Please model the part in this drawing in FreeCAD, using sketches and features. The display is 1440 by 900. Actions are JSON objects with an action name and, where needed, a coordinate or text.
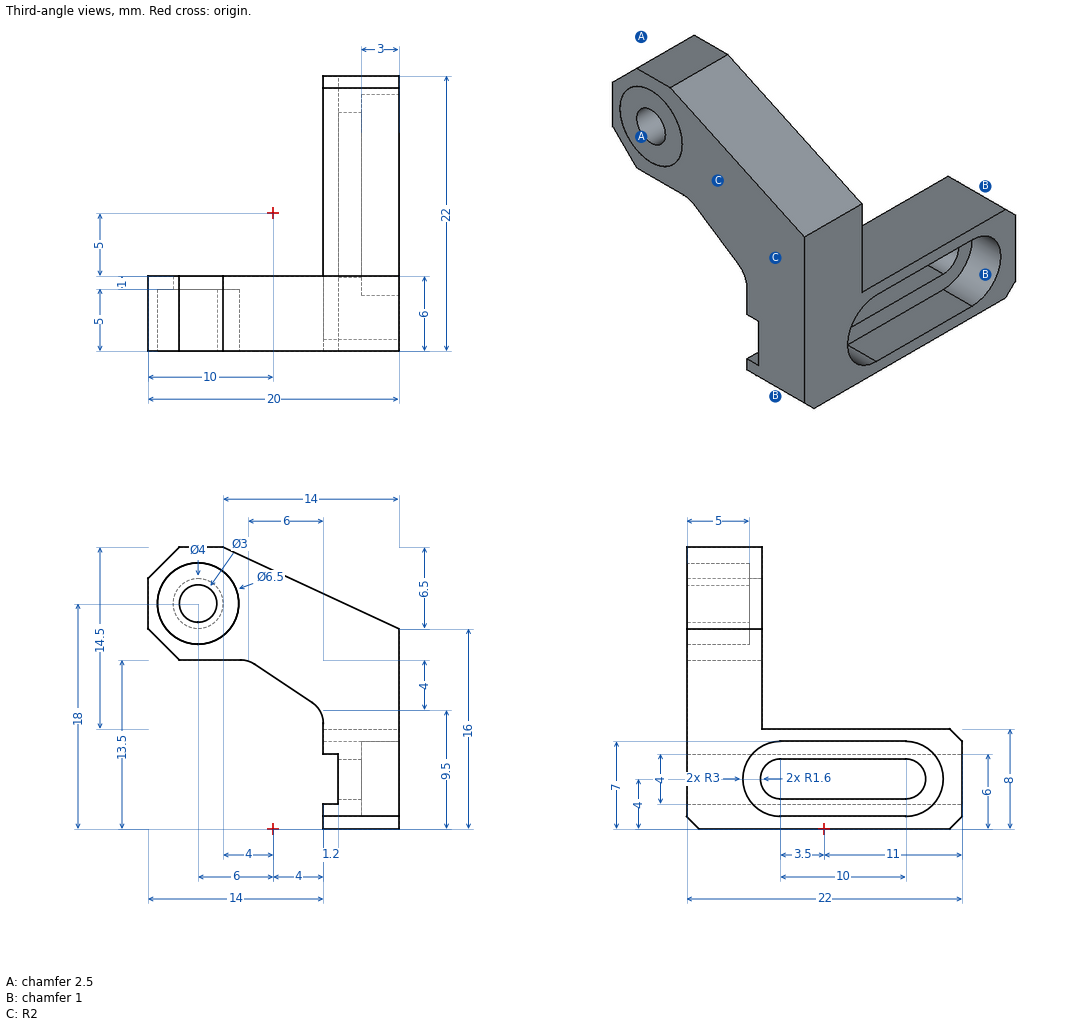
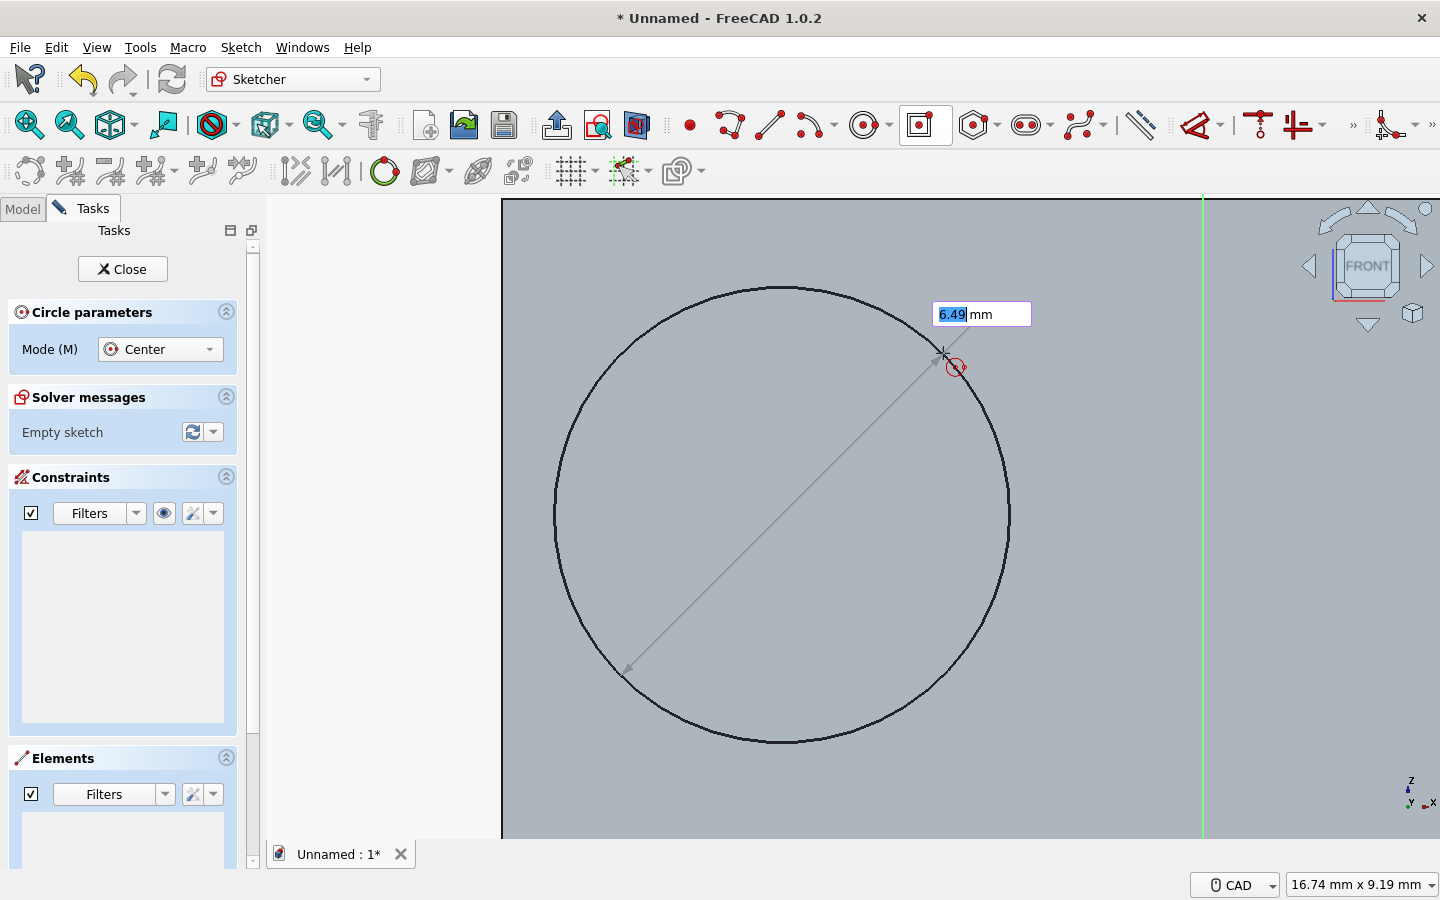
{"action": "type", "text": "6.5"}
{"action": "key", "text": "Return"}
{"action": "key", "text": "Escape"}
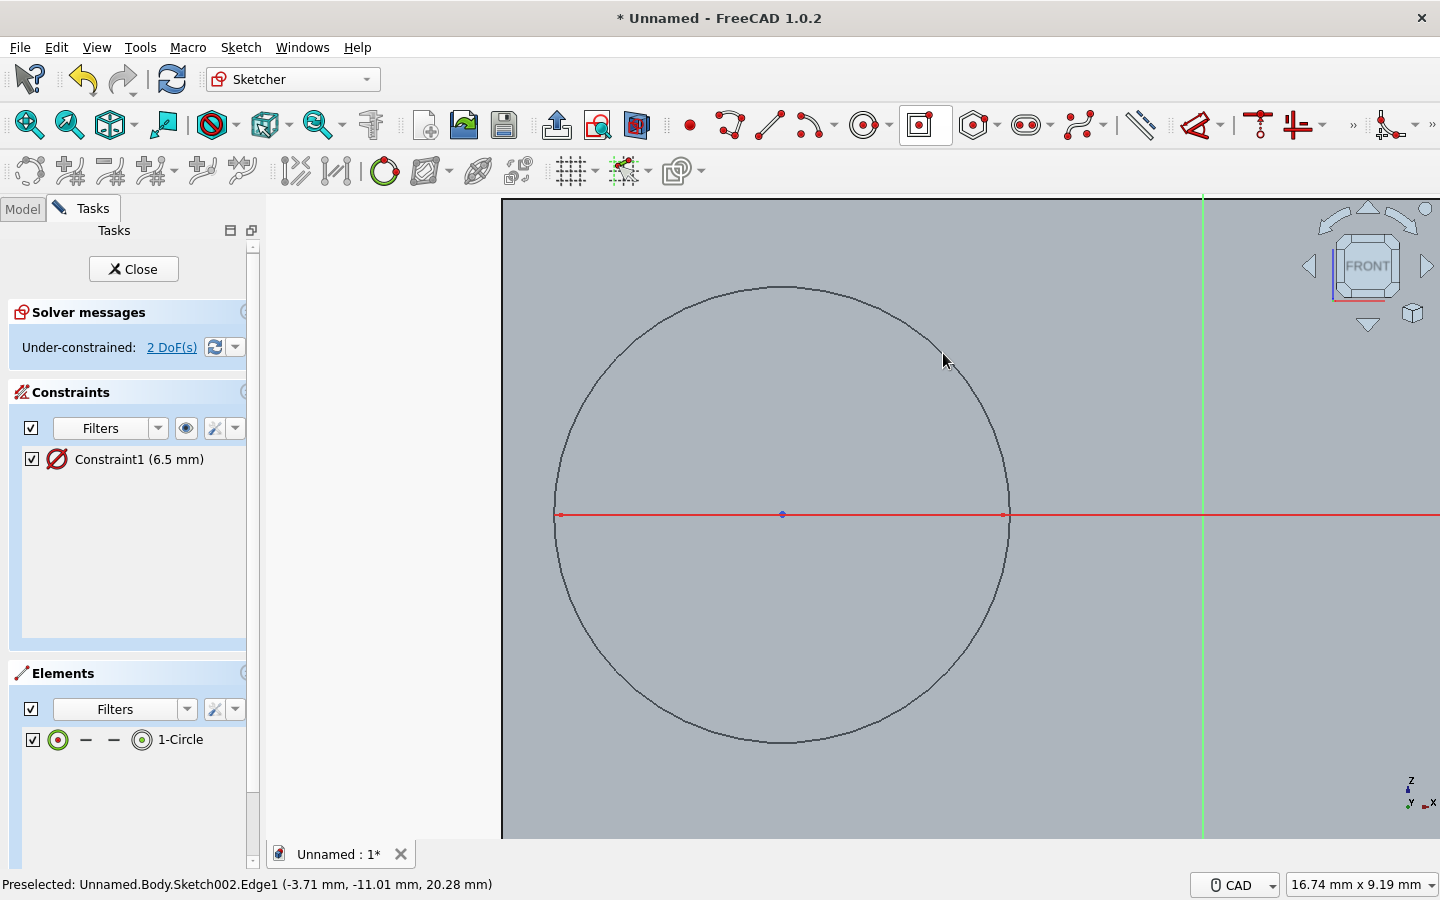
{"action": "left_click", "coordinate": [1196, 126]}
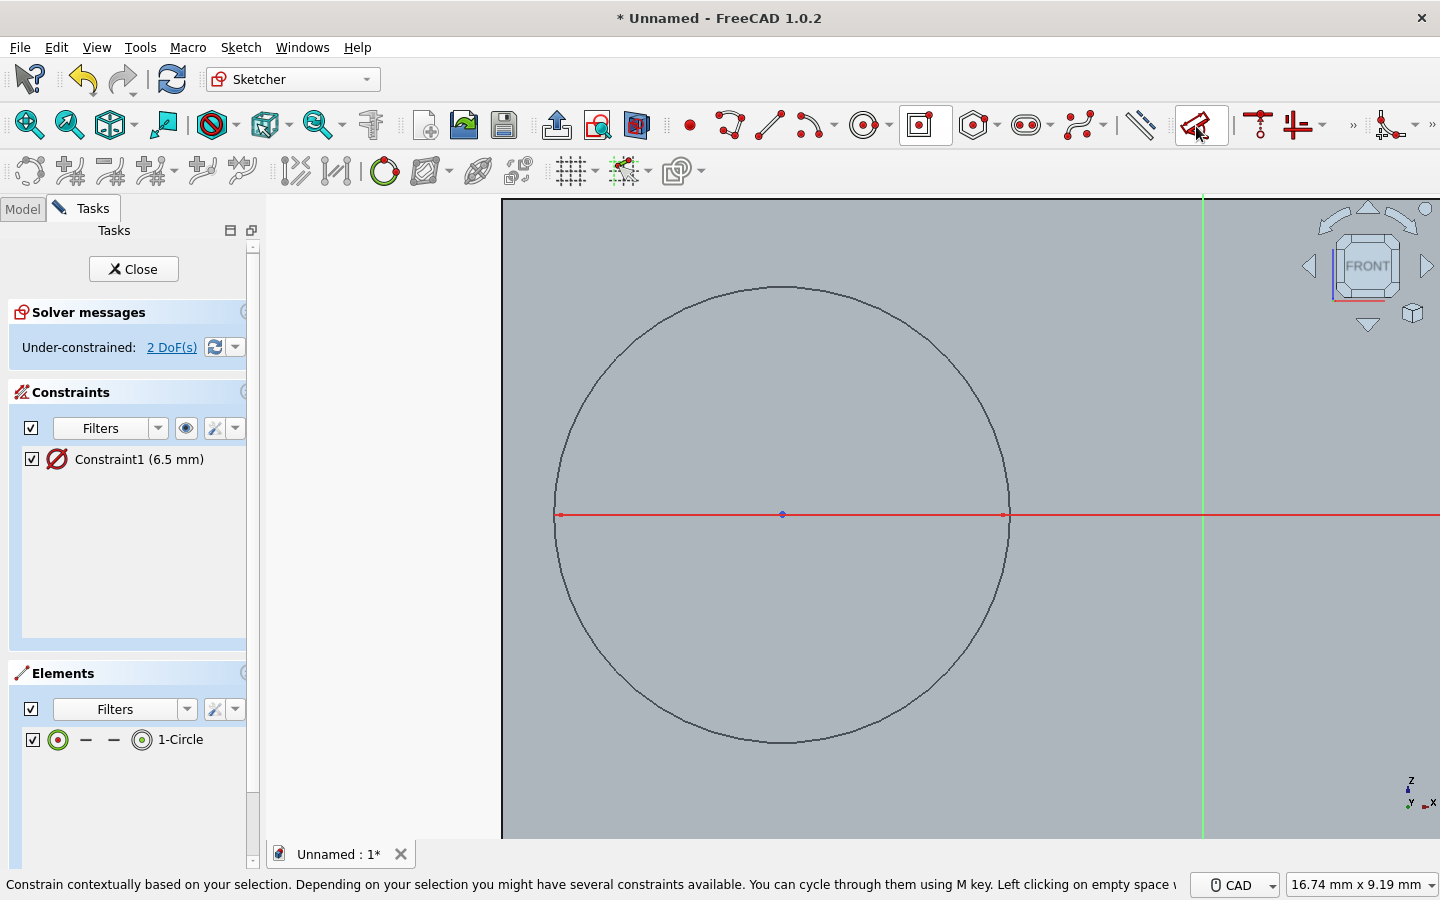
{"action": "left_click", "coordinate": [782, 515]}
{"action": "left_click", "coordinate": [993, 481]}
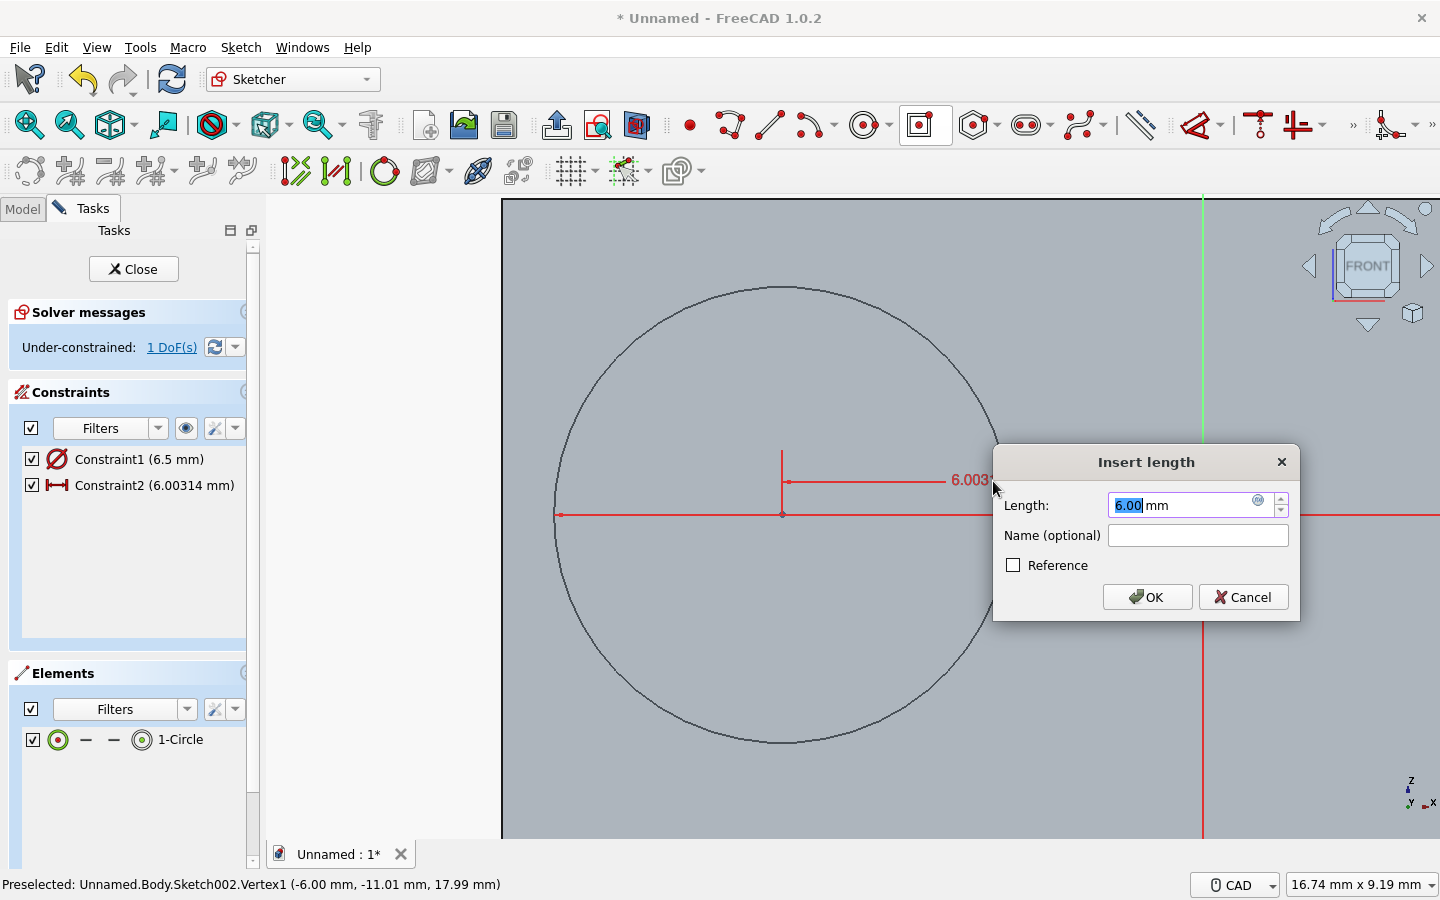
{"action": "type", "text": "6"}
{"action": "key", "text": "Return"}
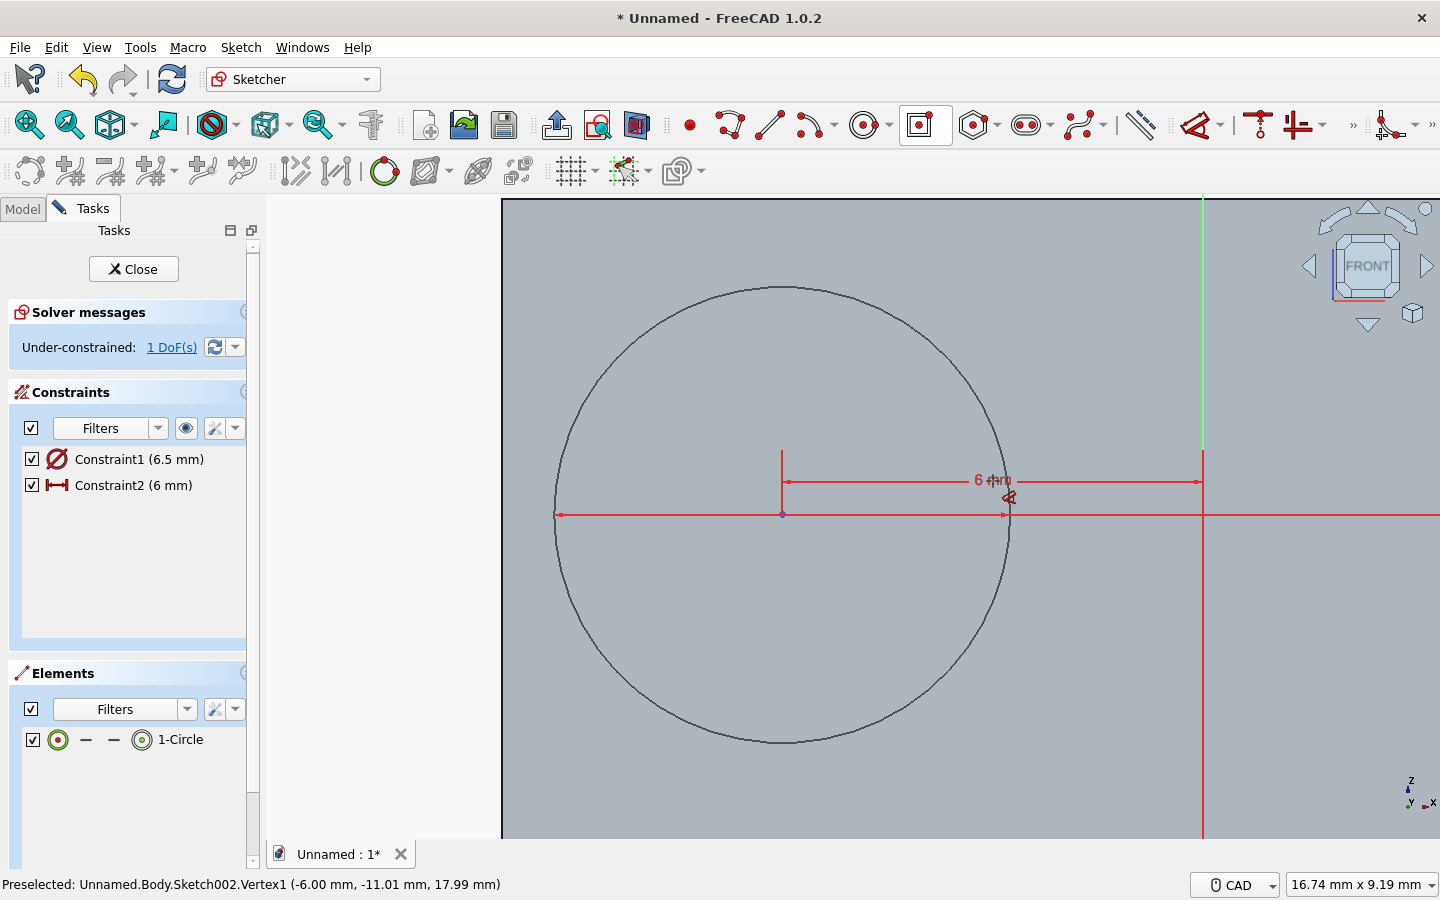
{"action": "left_click", "coordinate": [782, 515]}
{"action": "left_click", "coordinate": [1237, 663]}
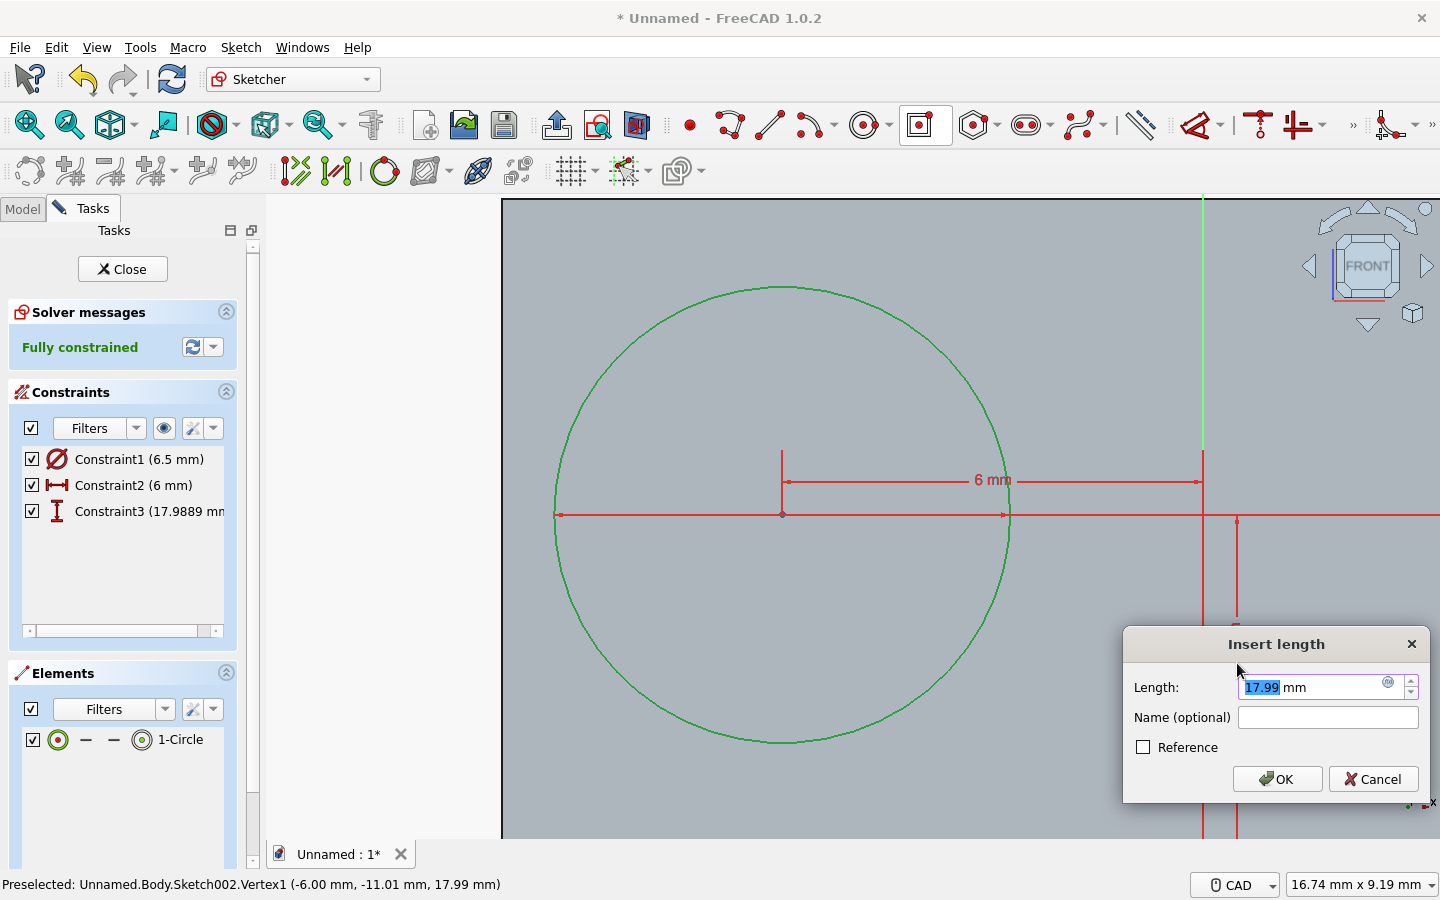
{"action": "type", "text": "18"}
{"action": "key", "text": "Return"}
{"action": "key", "text": "Escape"}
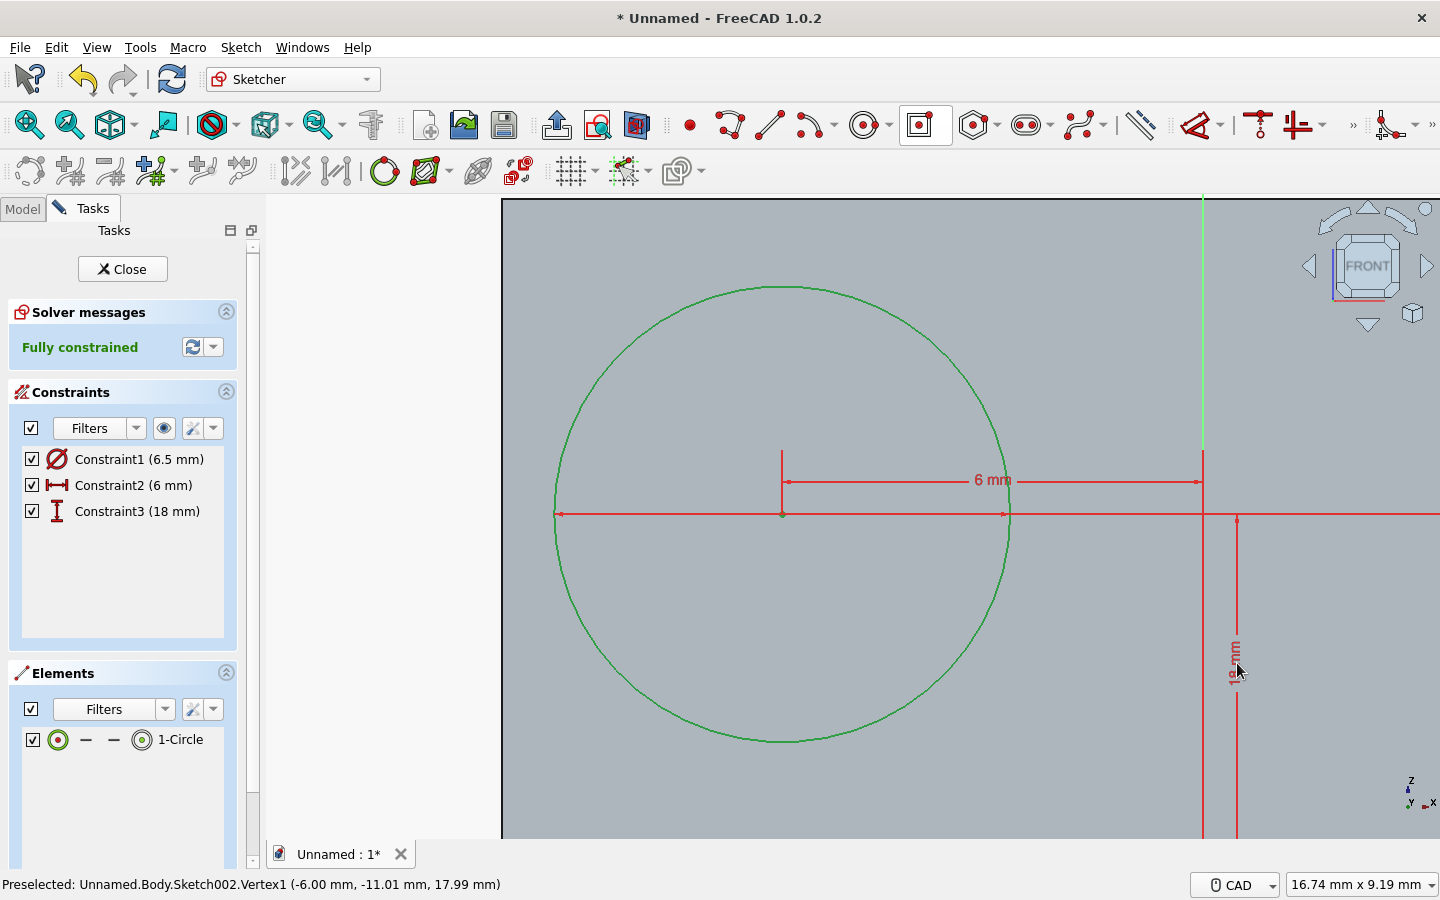
{"action": "left_click", "coordinate": [123, 269]}